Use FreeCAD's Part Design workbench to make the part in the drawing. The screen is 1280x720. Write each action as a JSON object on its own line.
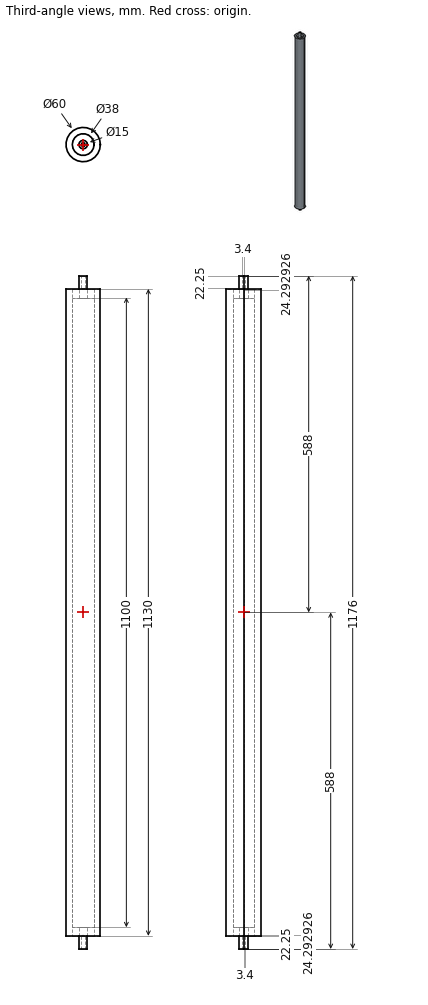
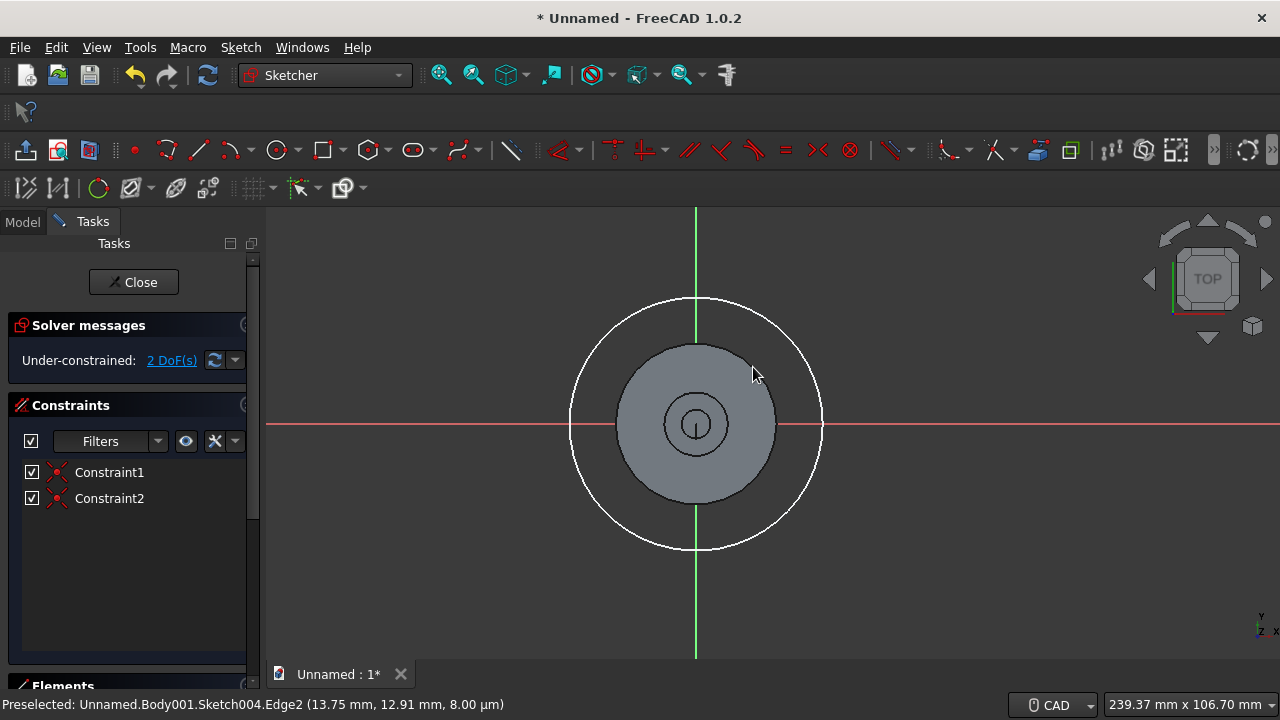
{"action": "left_click", "coordinate": [558, 150]}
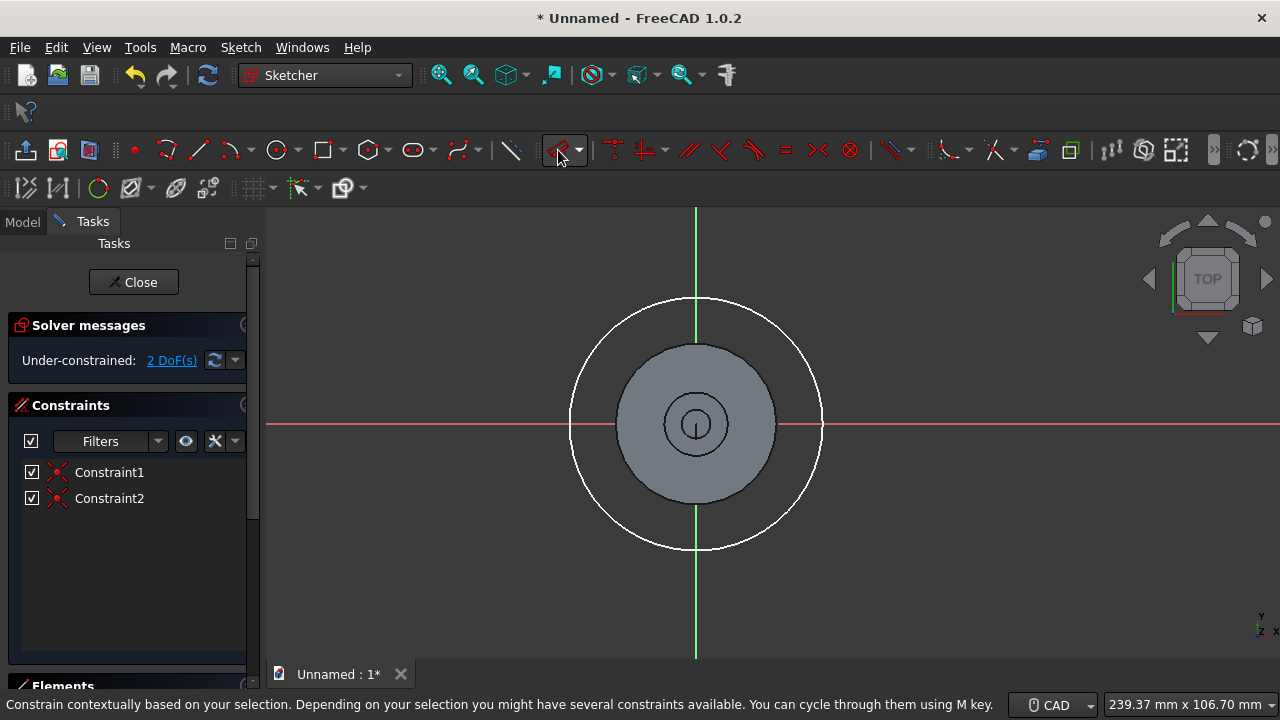
{"action": "left_click", "coordinate": [785, 334]}
{"action": "left_click", "coordinate": [807, 311]}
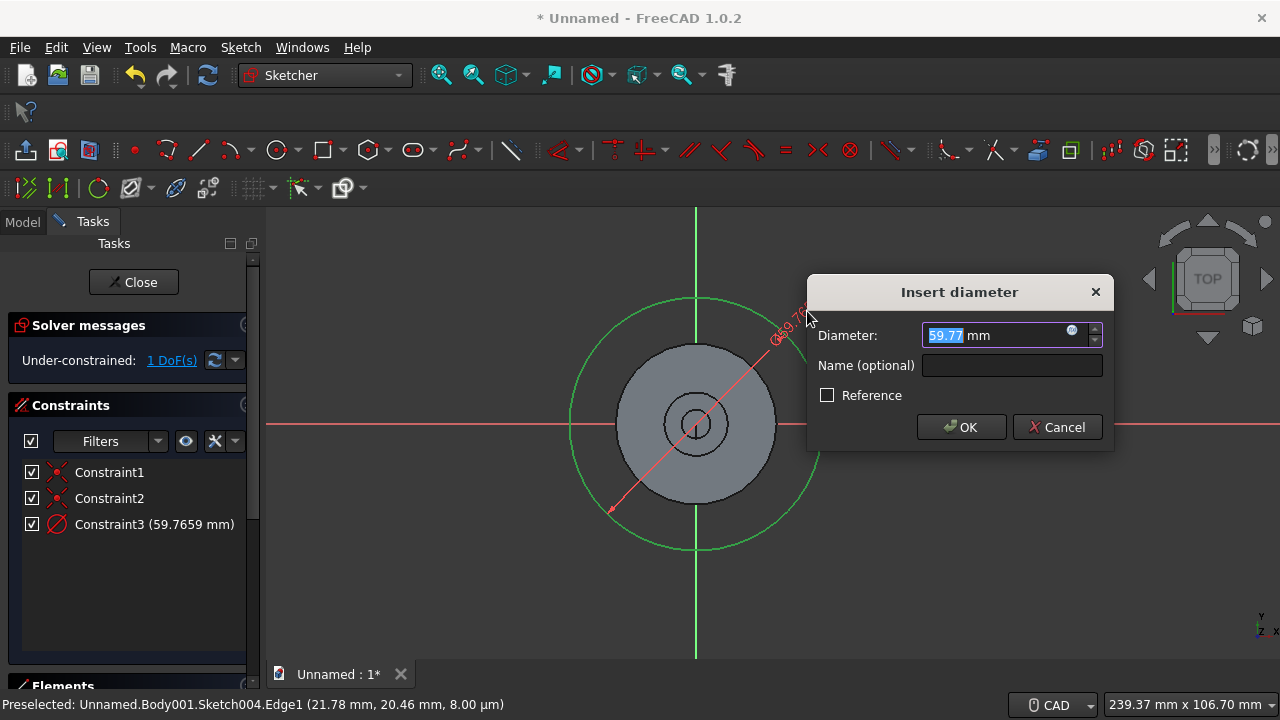
{"action": "type", "text": "60"}
{"action": "key", "text": "Return"}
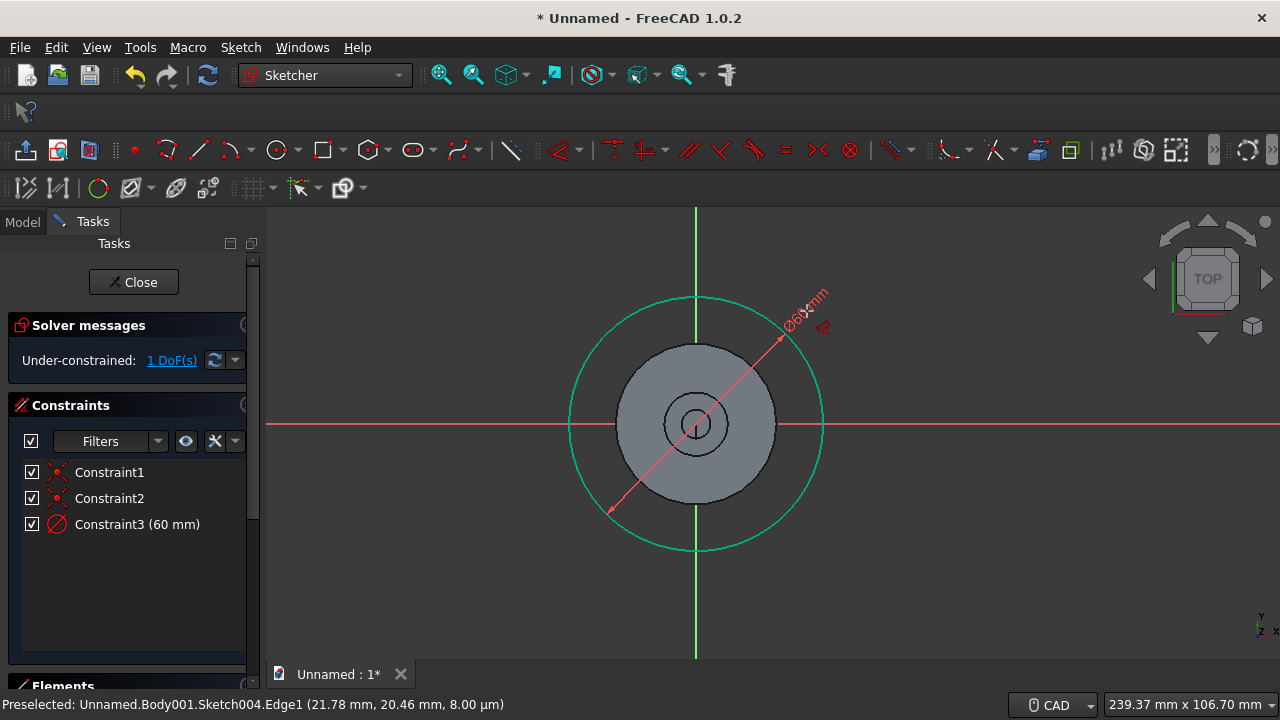
{"action": "left_click", "coordinate": [752, 367]}
{"action": "left_click", "coordinate": [774, 344]}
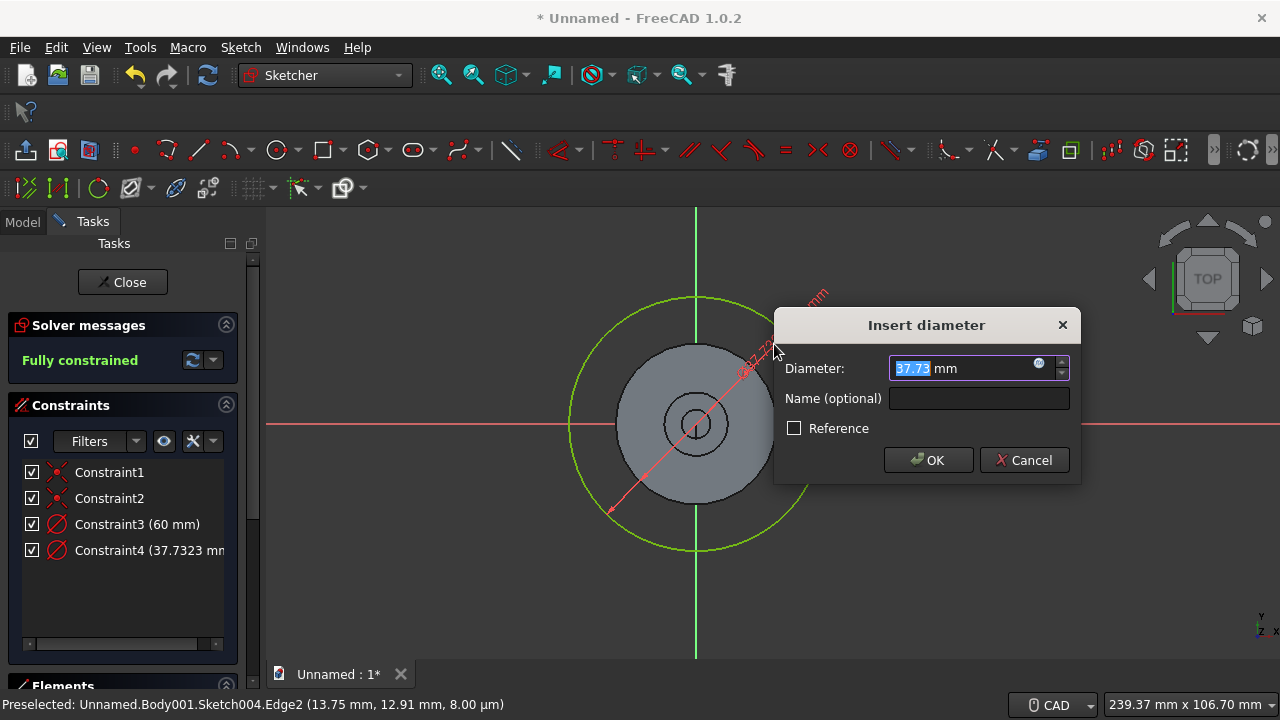
{"action": "type", "text": "38"}
{"action": "key", "text": "Return"}
{"action": "key", "text": "Escape"}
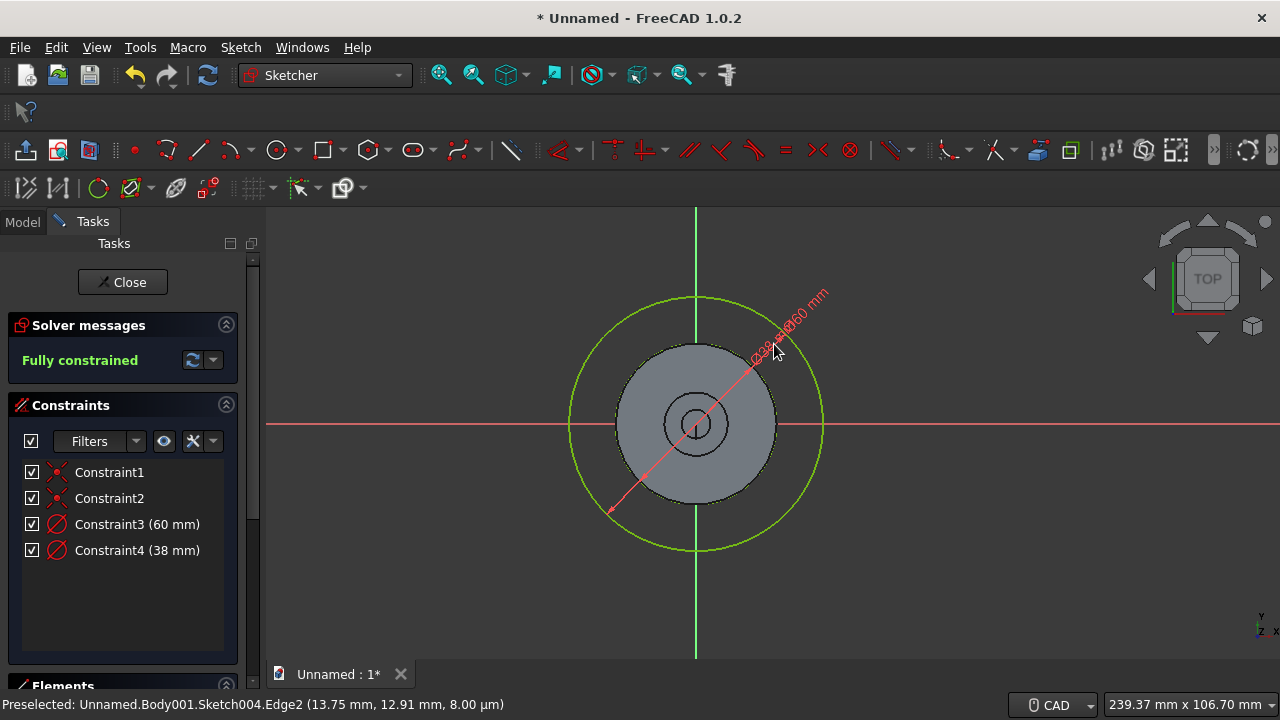
{"action": "left_click", "coordinate": [123, 282]}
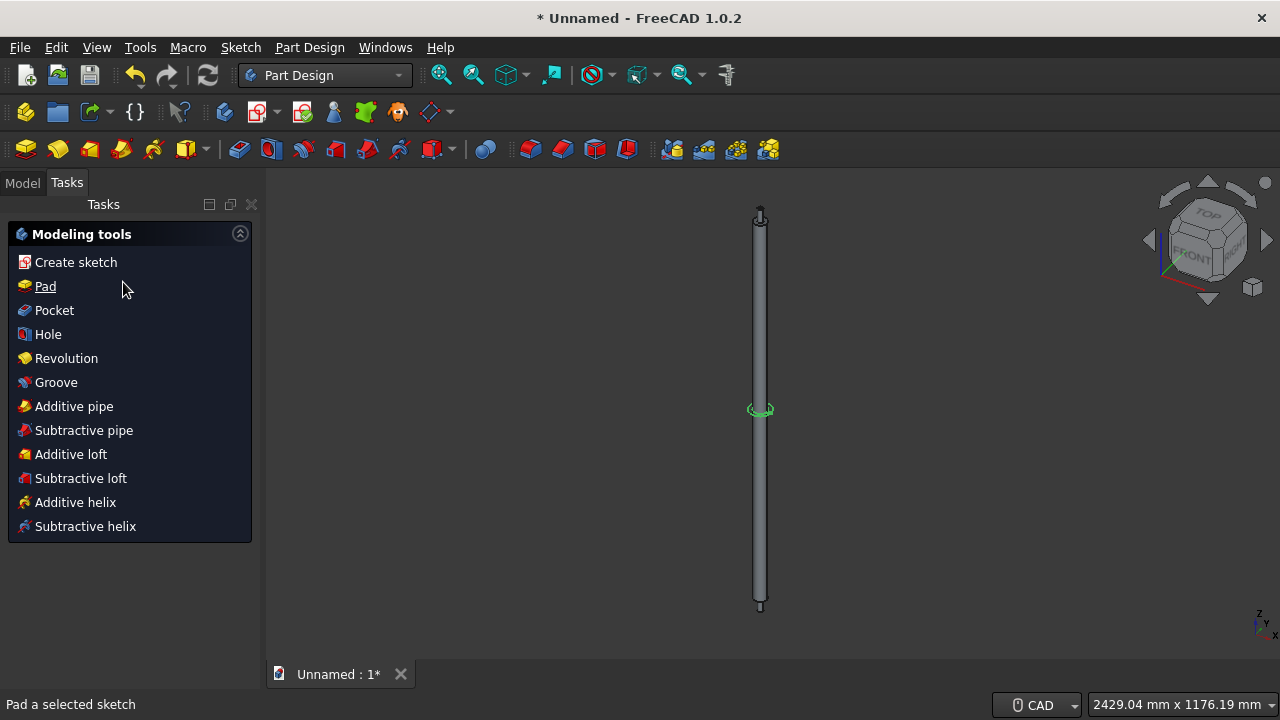
{"action": "left_click", "coordinate": [26, 150]}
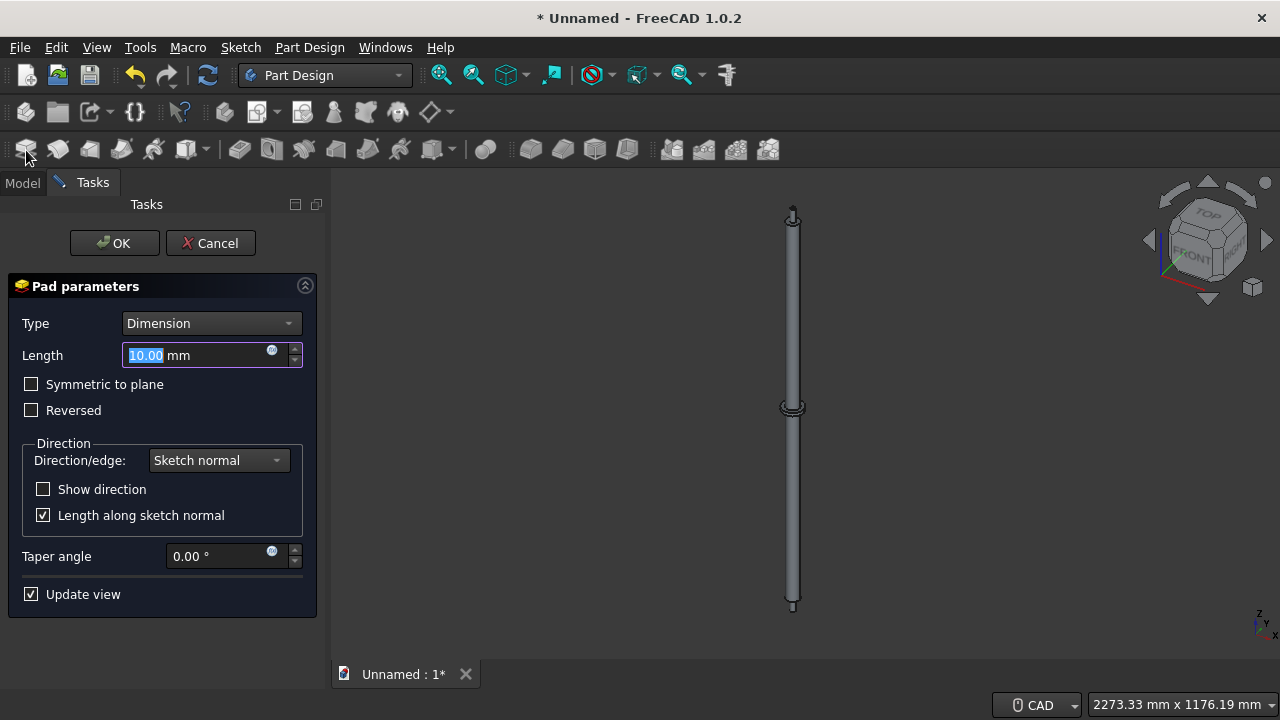
{"action": "type", "text": "1130"}
{"action": "key", "text": "Tab"}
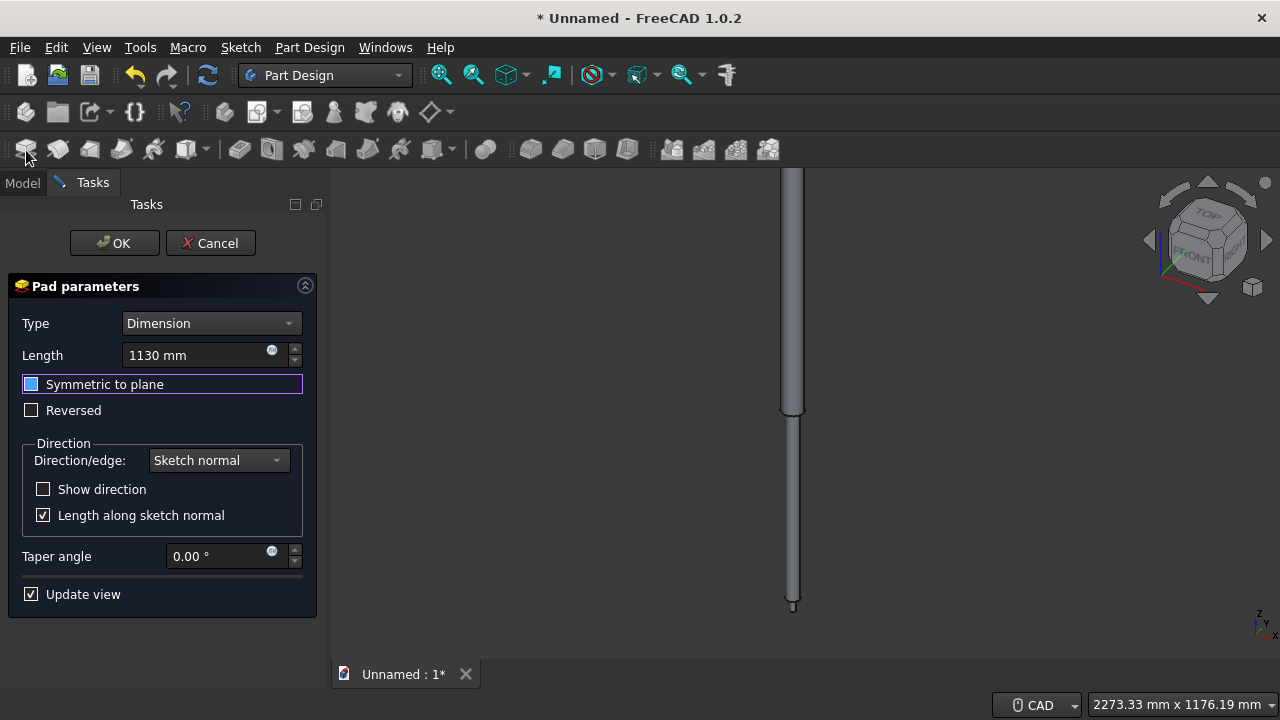
{"action": "left_click", "coordinate": [30, 384]}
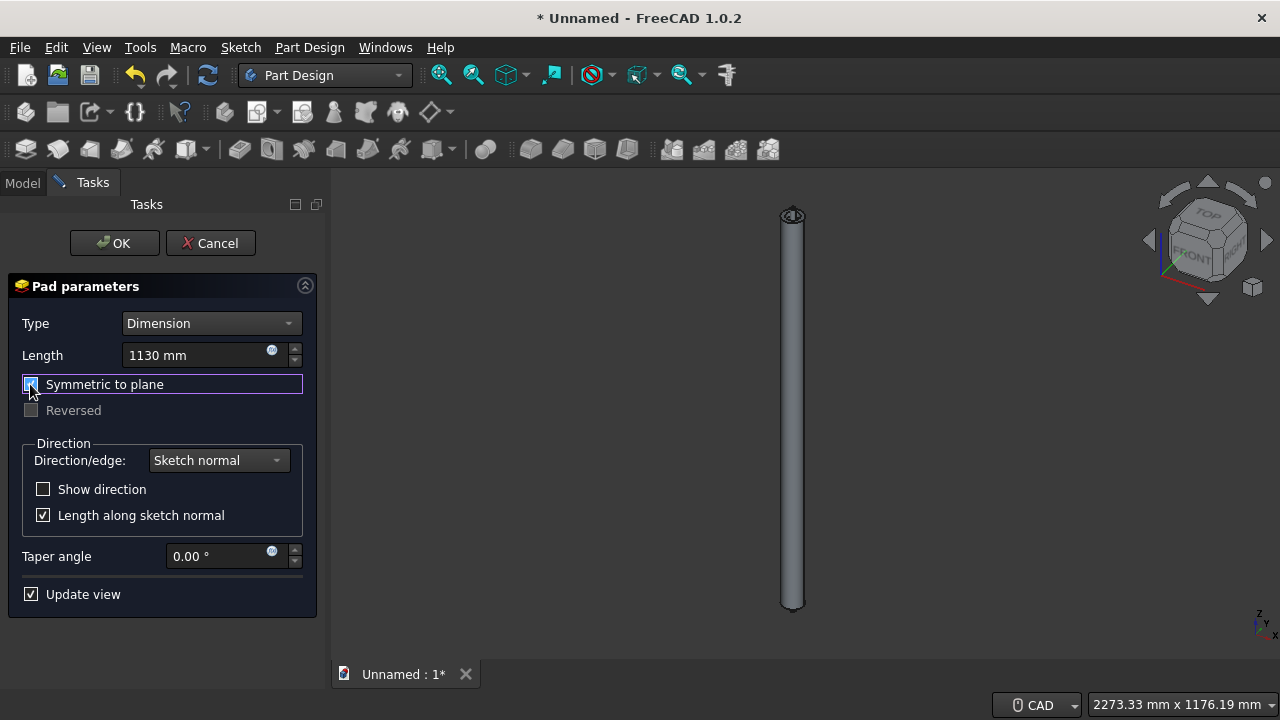
{"action": "left_click", "coordinate": [115, 243]}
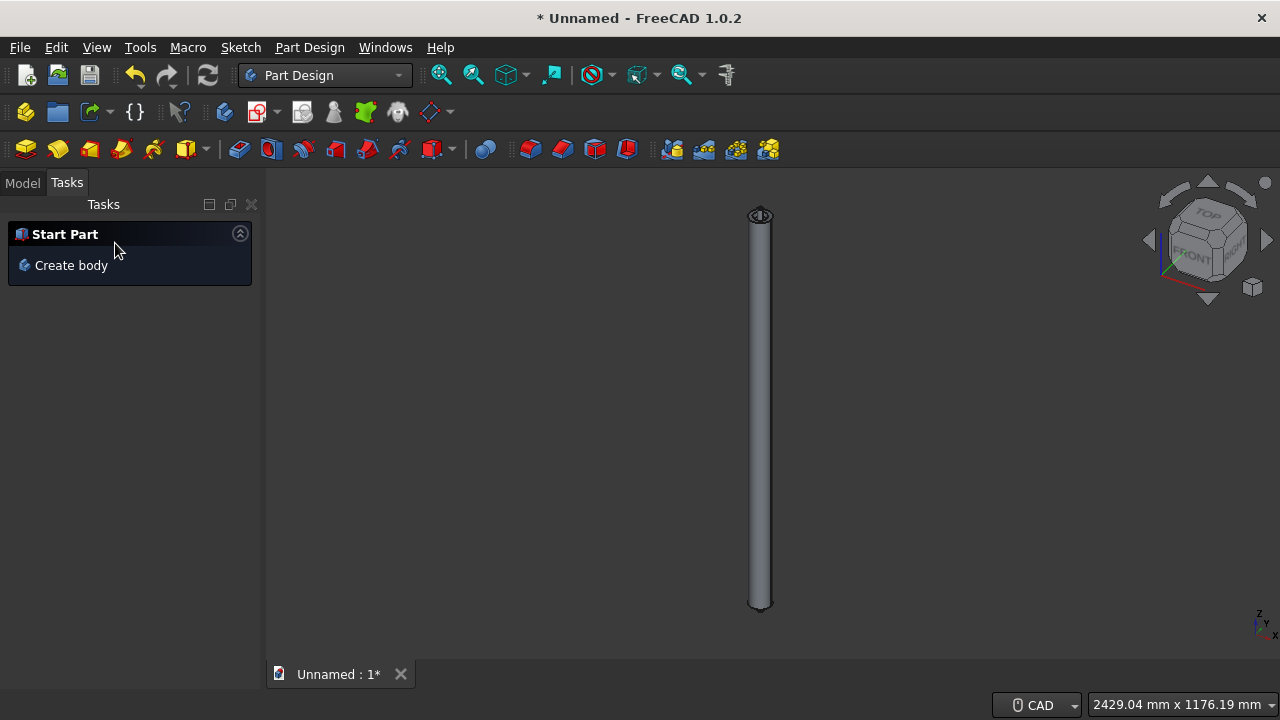
{"action": "key", "text": "0"}